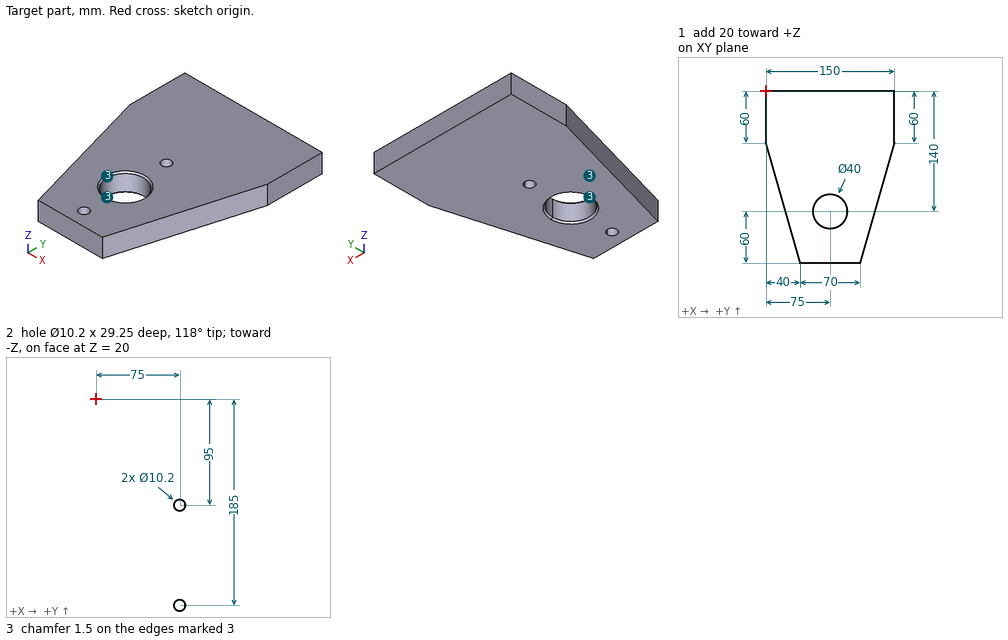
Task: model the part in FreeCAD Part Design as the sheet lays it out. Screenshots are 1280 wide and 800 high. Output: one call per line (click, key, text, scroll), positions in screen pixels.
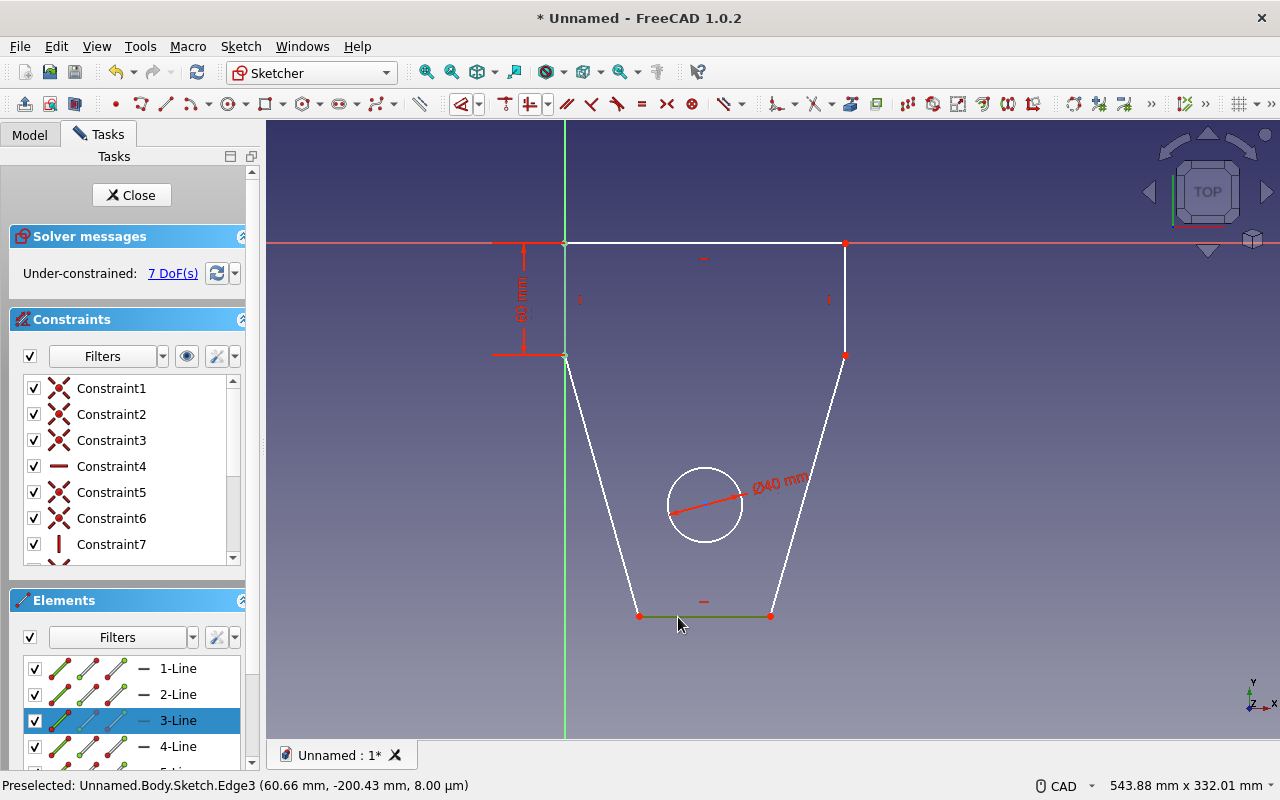
key(l)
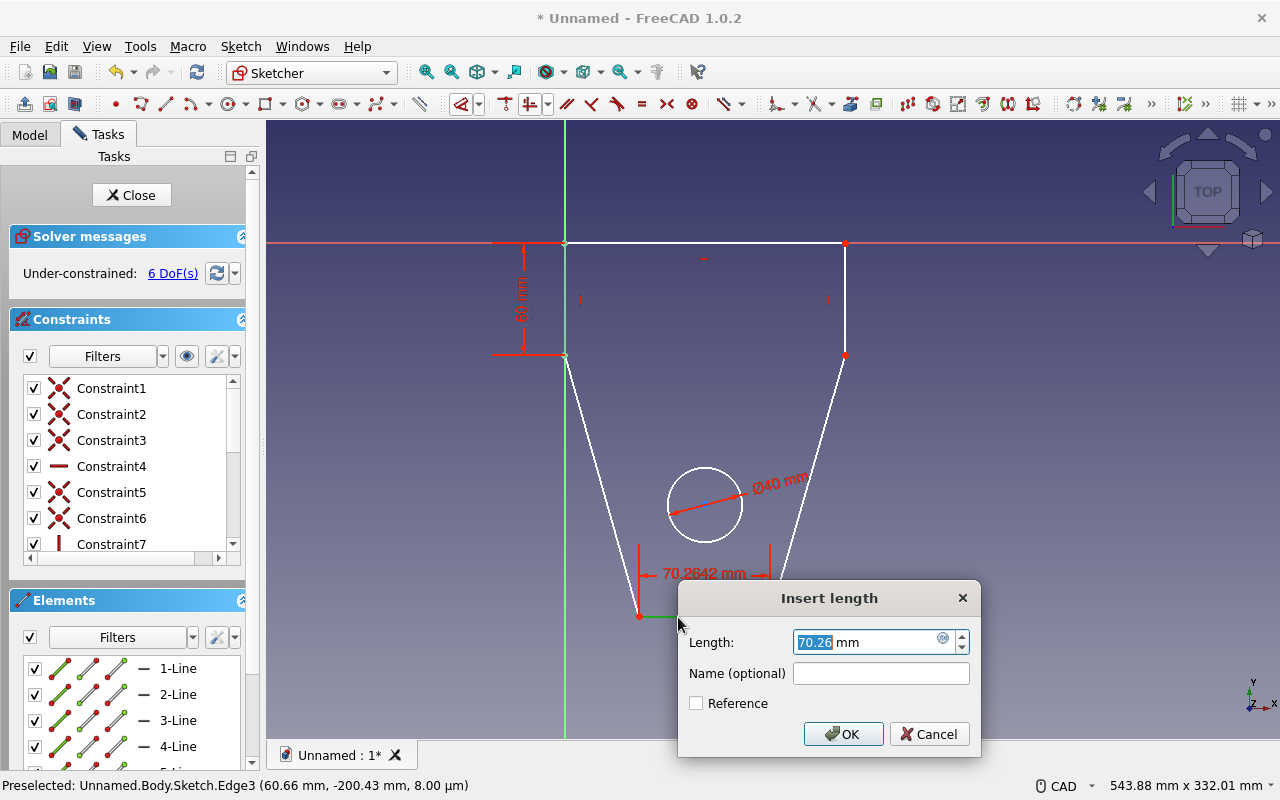
text(70)
key(Return)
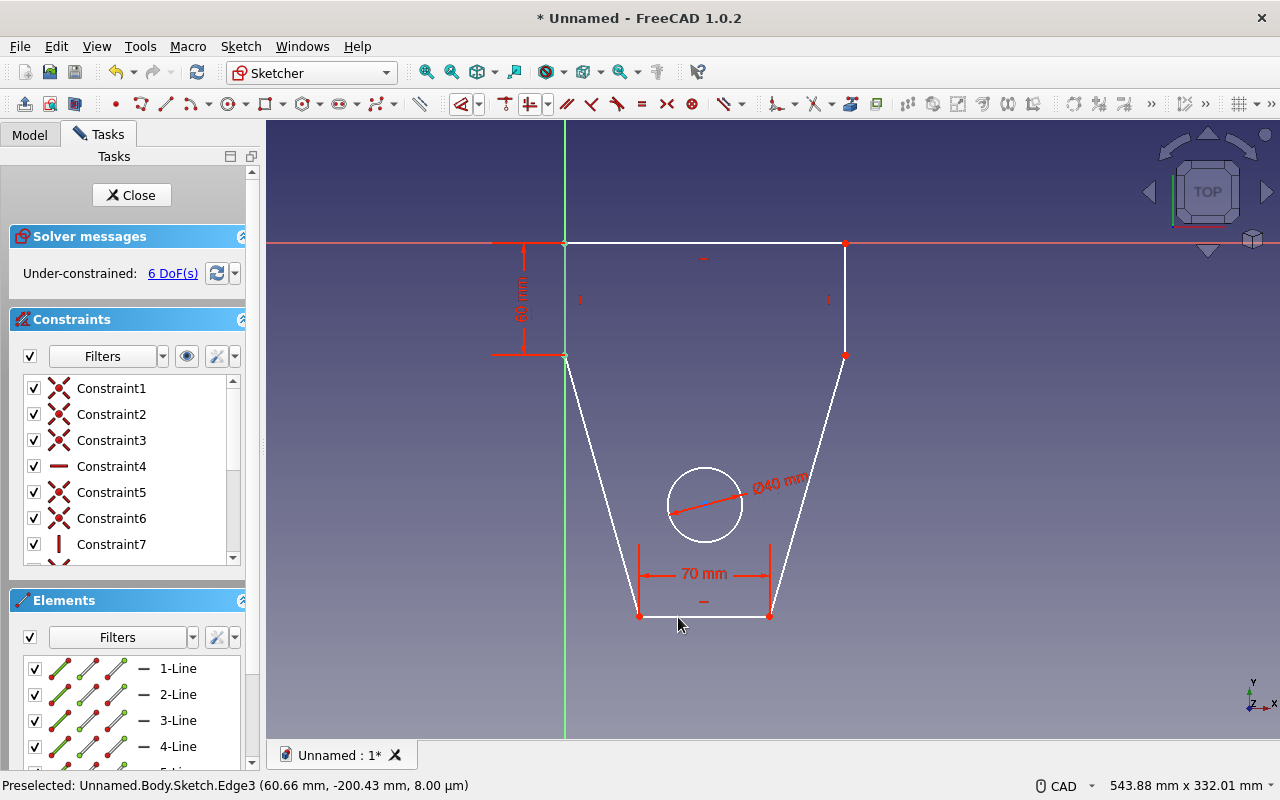
click(845, 322)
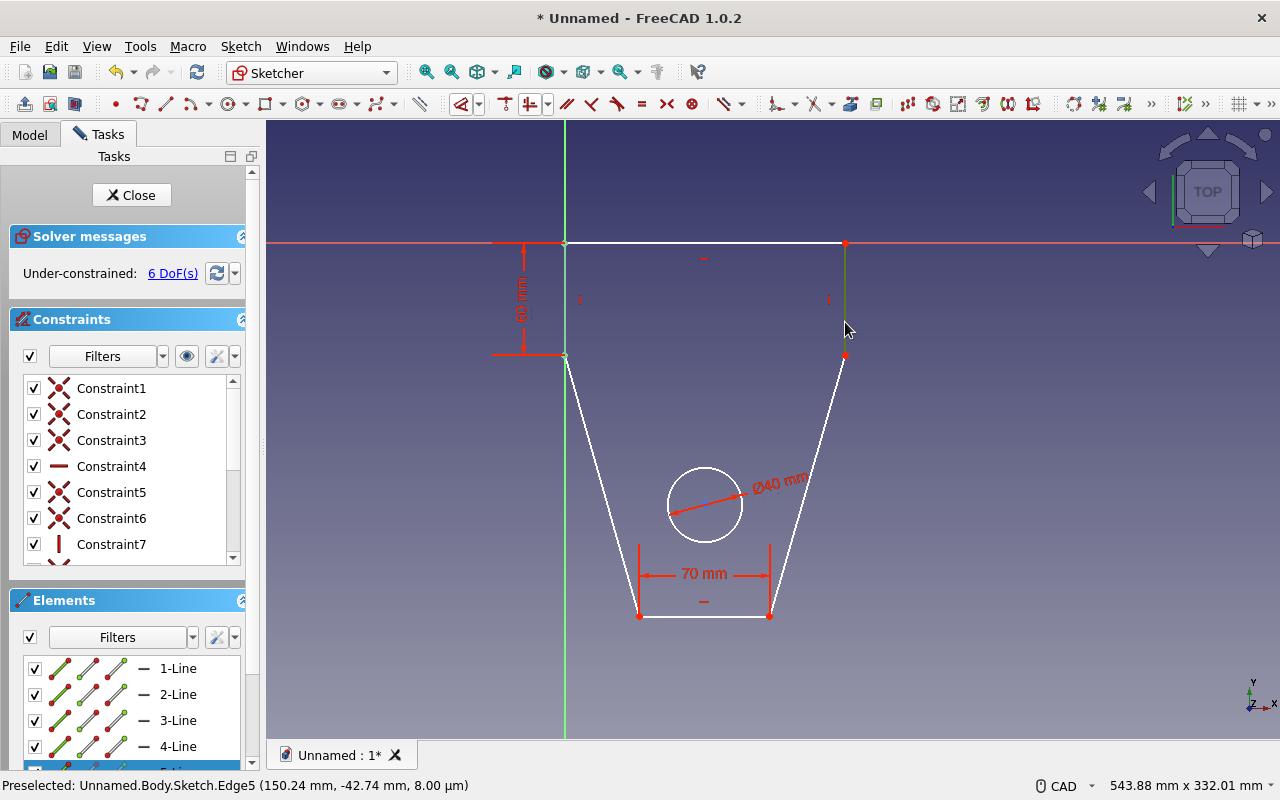
key(i)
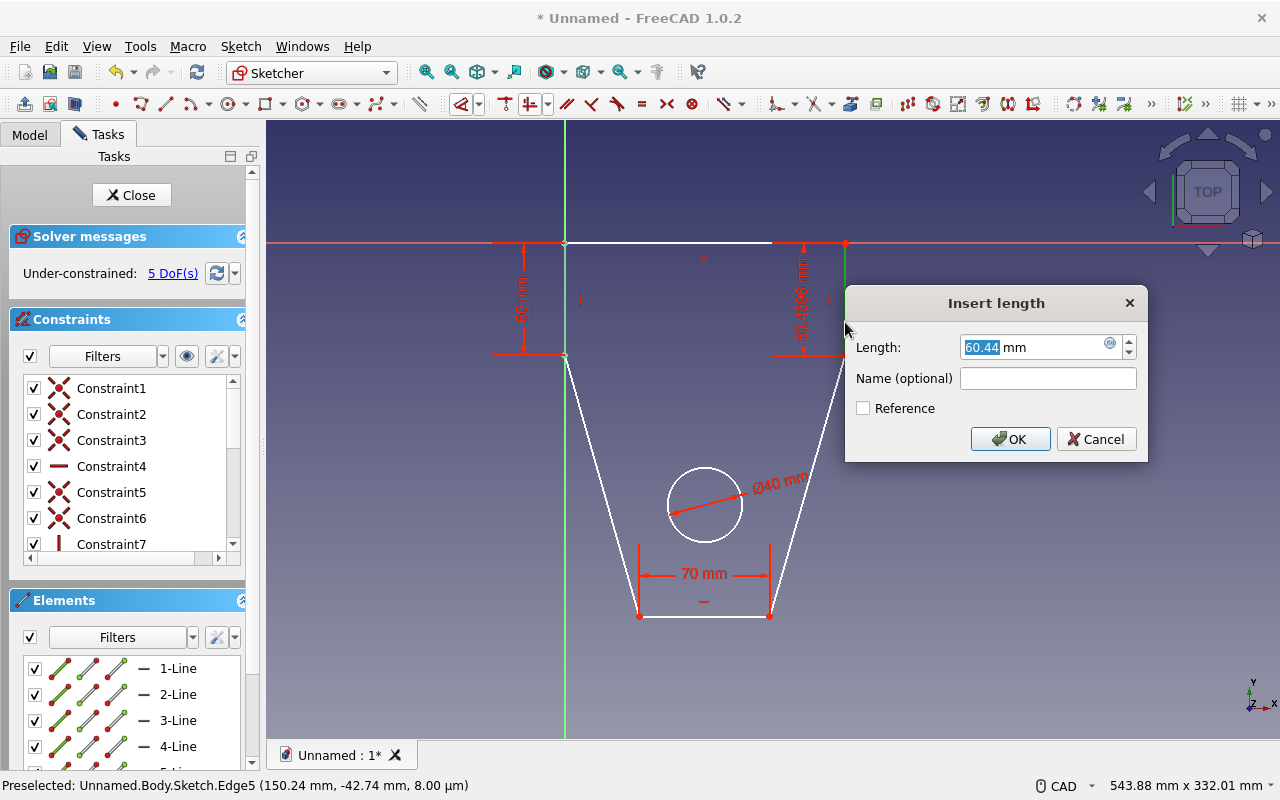
text(60)
key(Return)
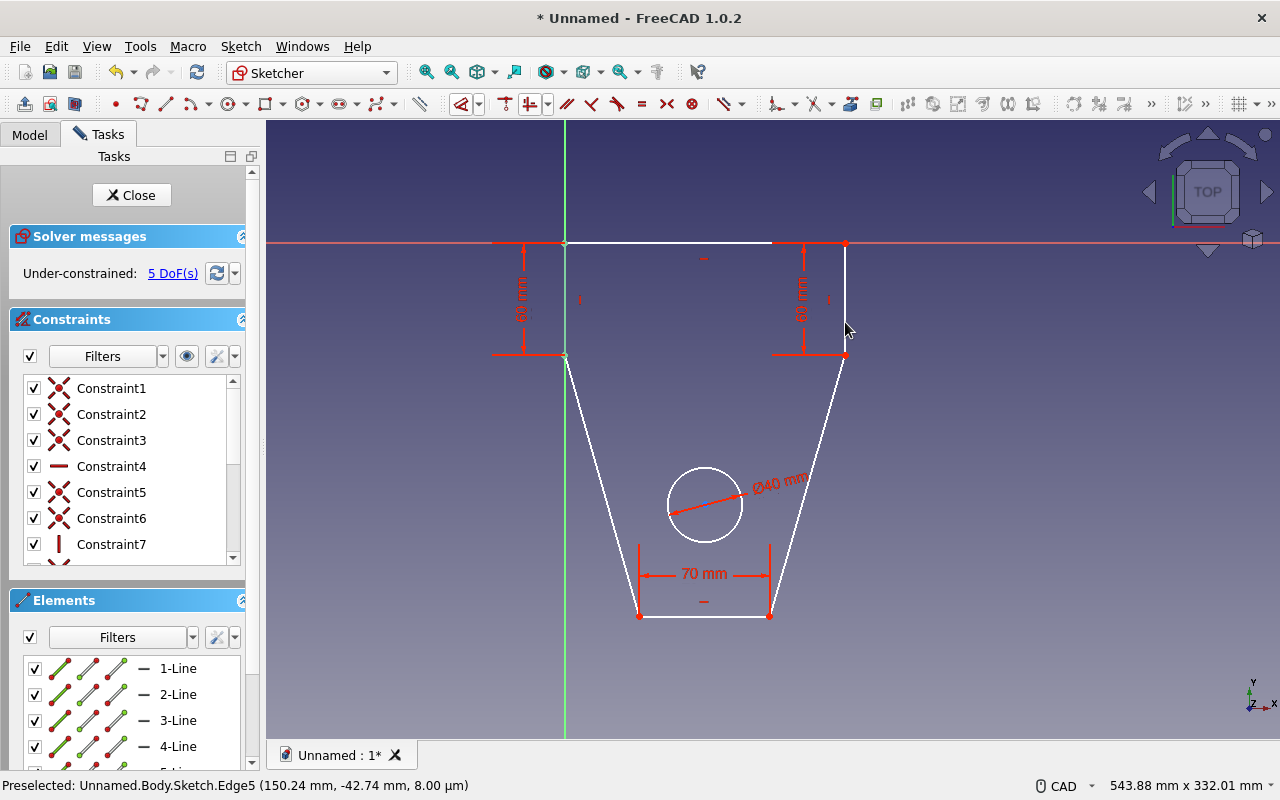
click(705, 505)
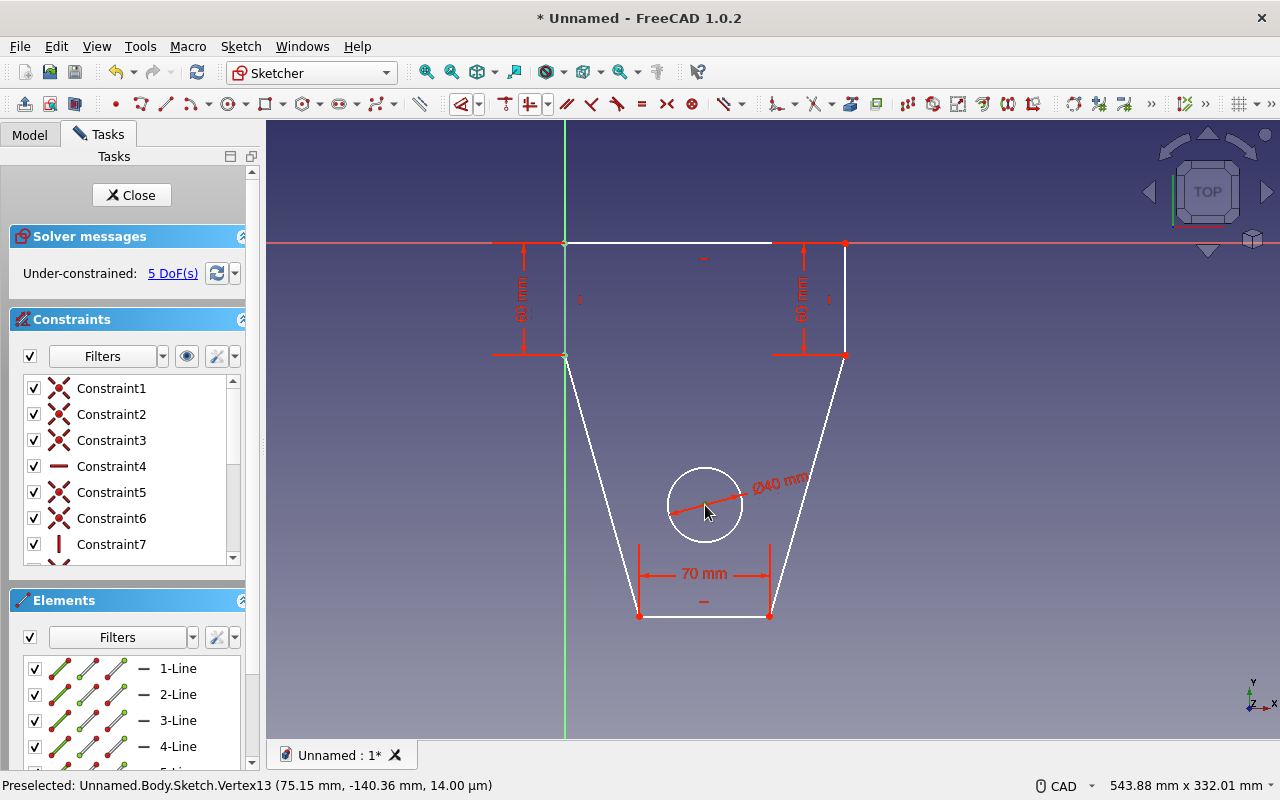
click(478, 104)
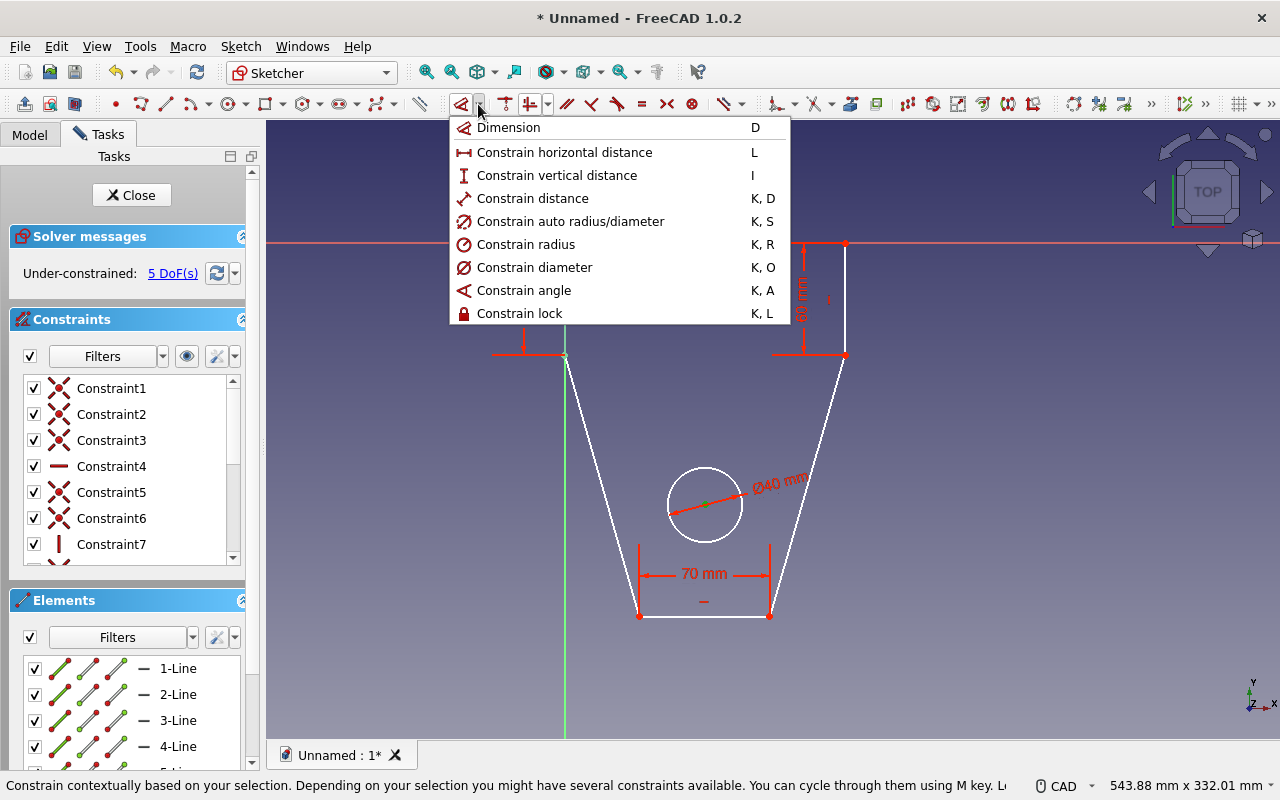
click(620, 152)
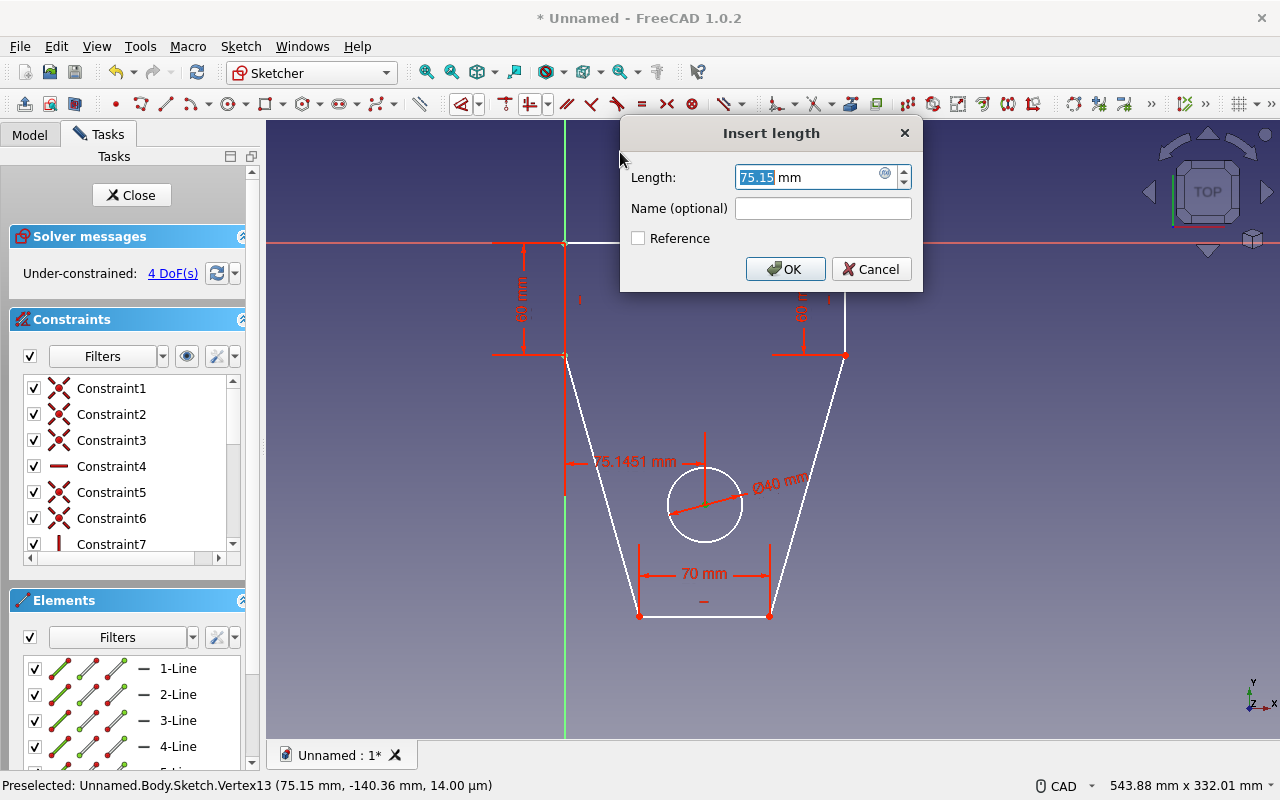
text(75)
key(Return)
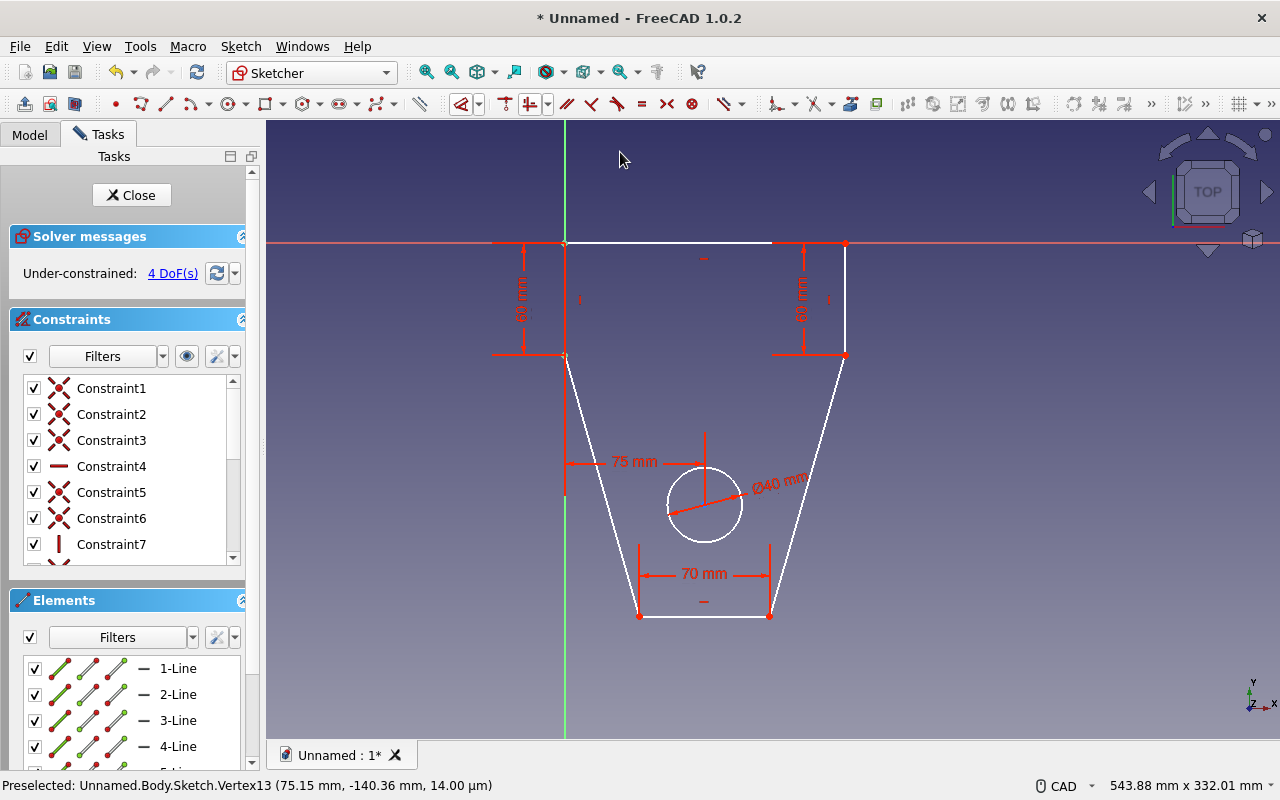
click(761, 243)